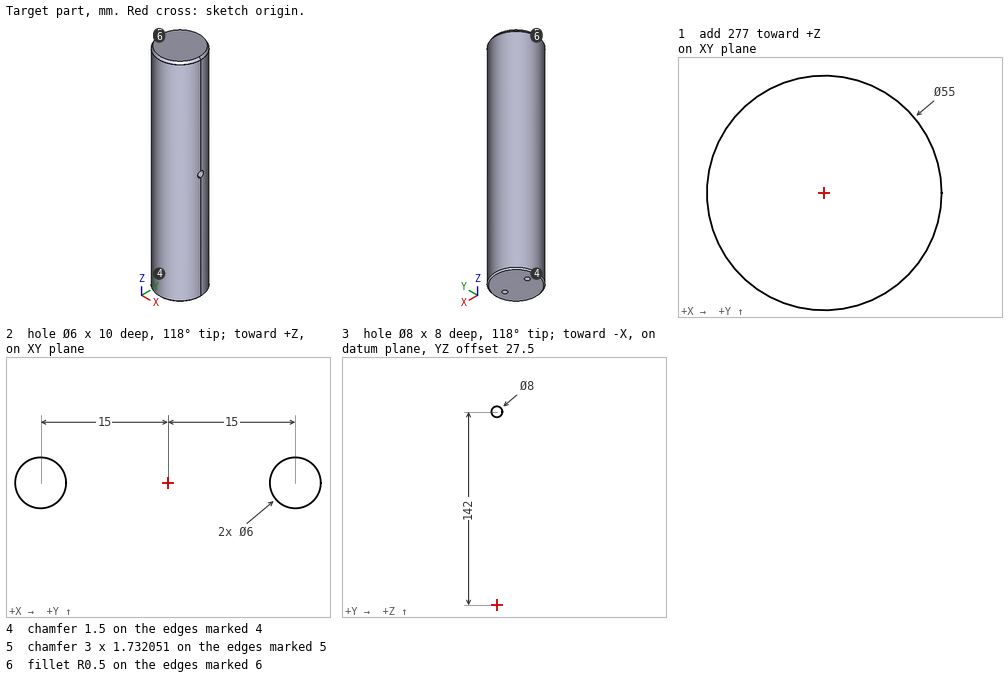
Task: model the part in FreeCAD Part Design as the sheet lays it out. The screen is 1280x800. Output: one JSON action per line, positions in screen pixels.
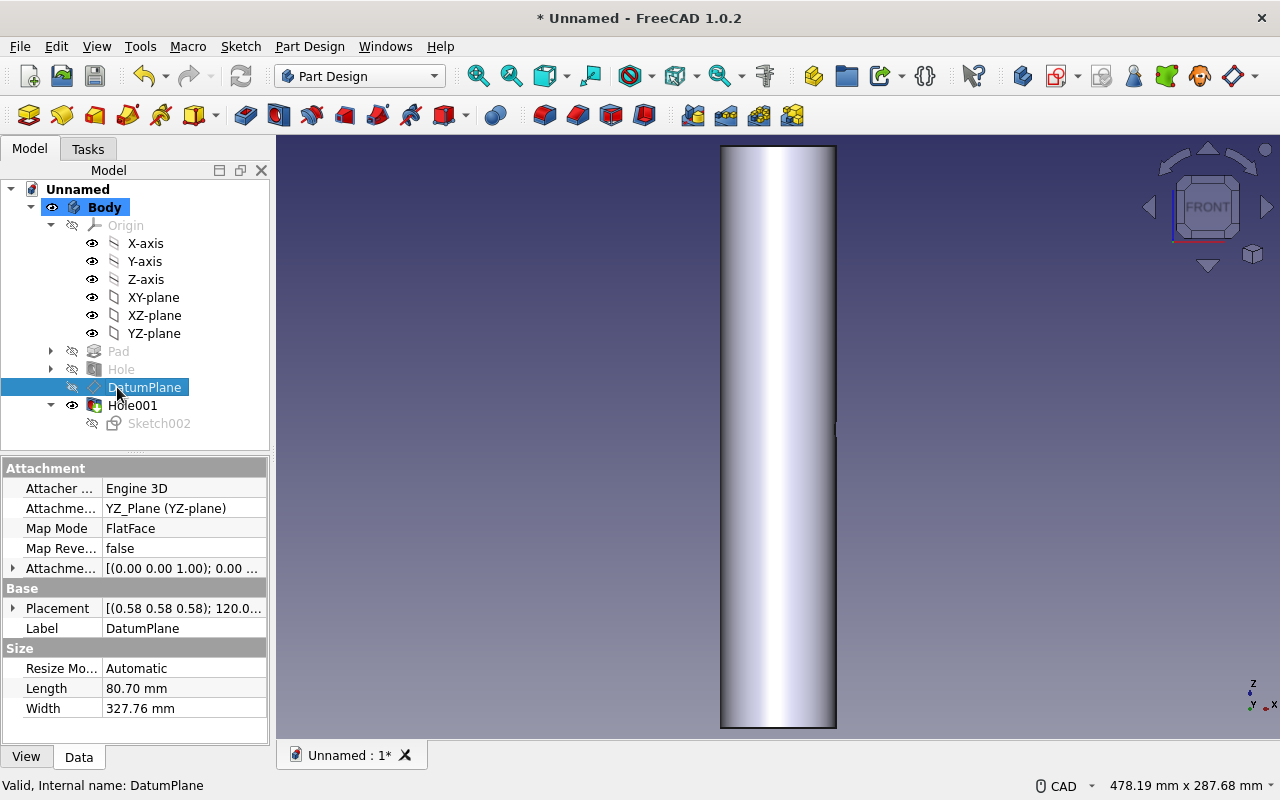
{"action": "key", "text": "3"}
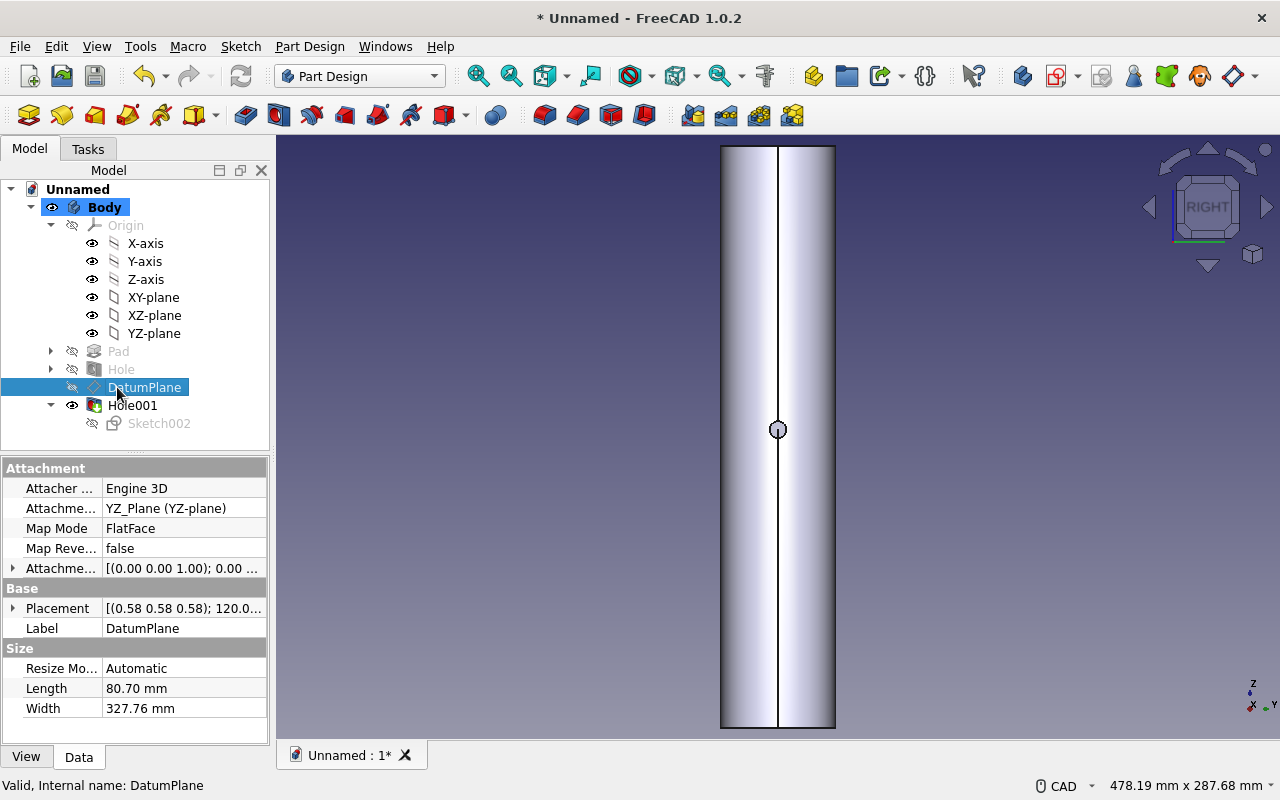
{"action": "key", "text": "5"}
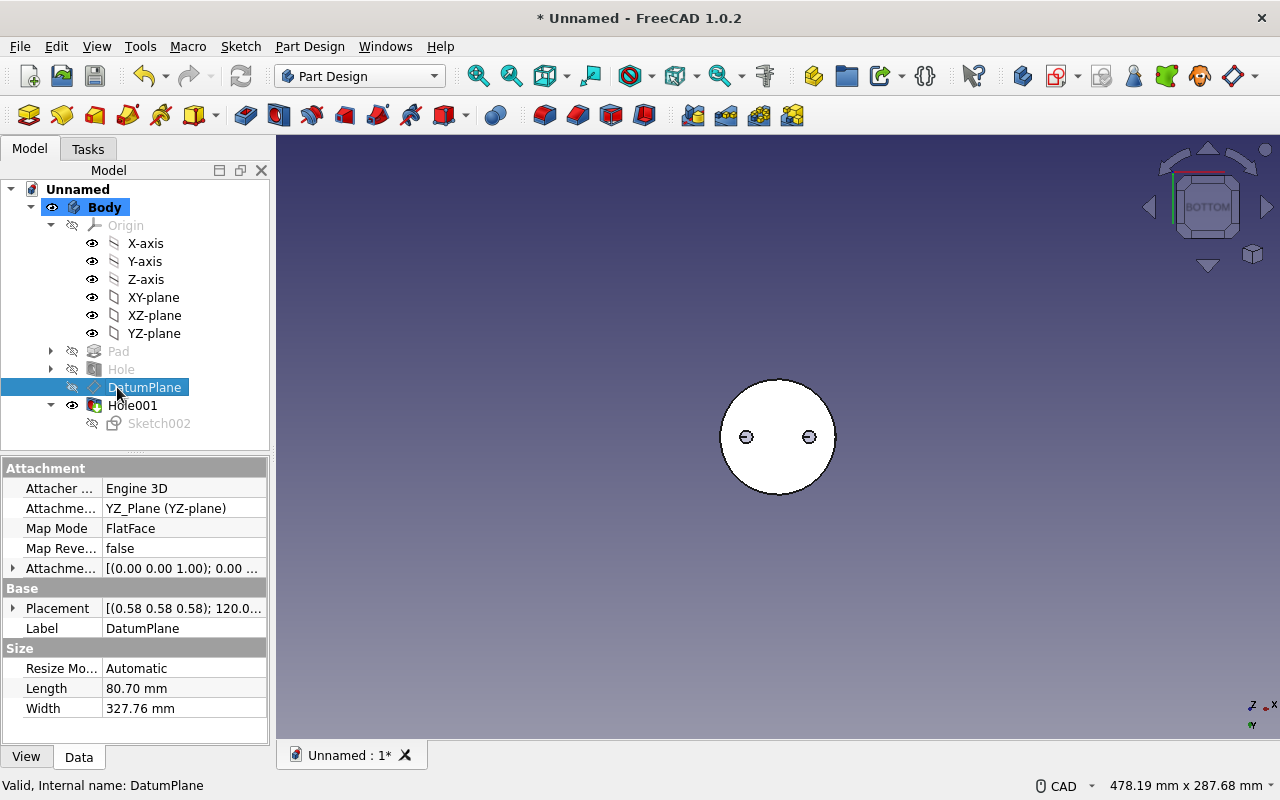
{"action": "left_click", "coordinate": [479, 76]}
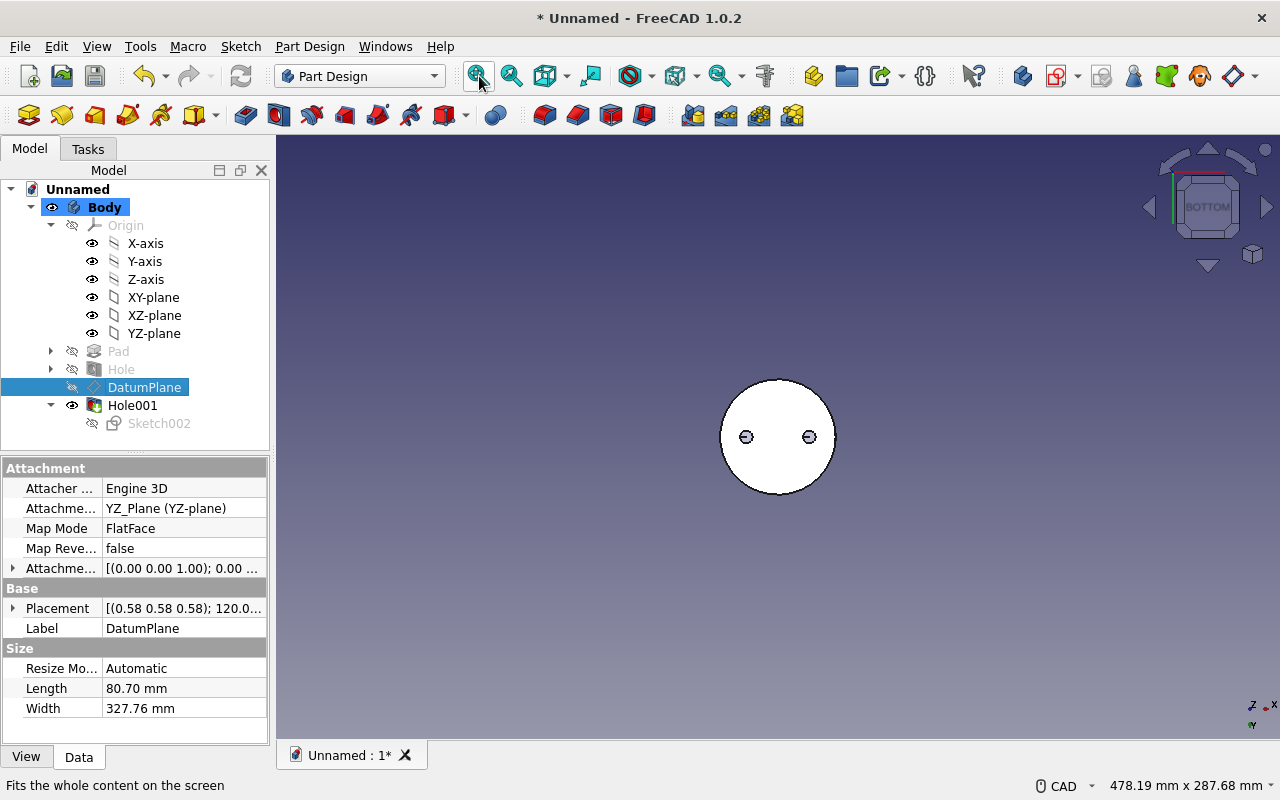
{"action": "left_click", "coordinate": [731, 470]}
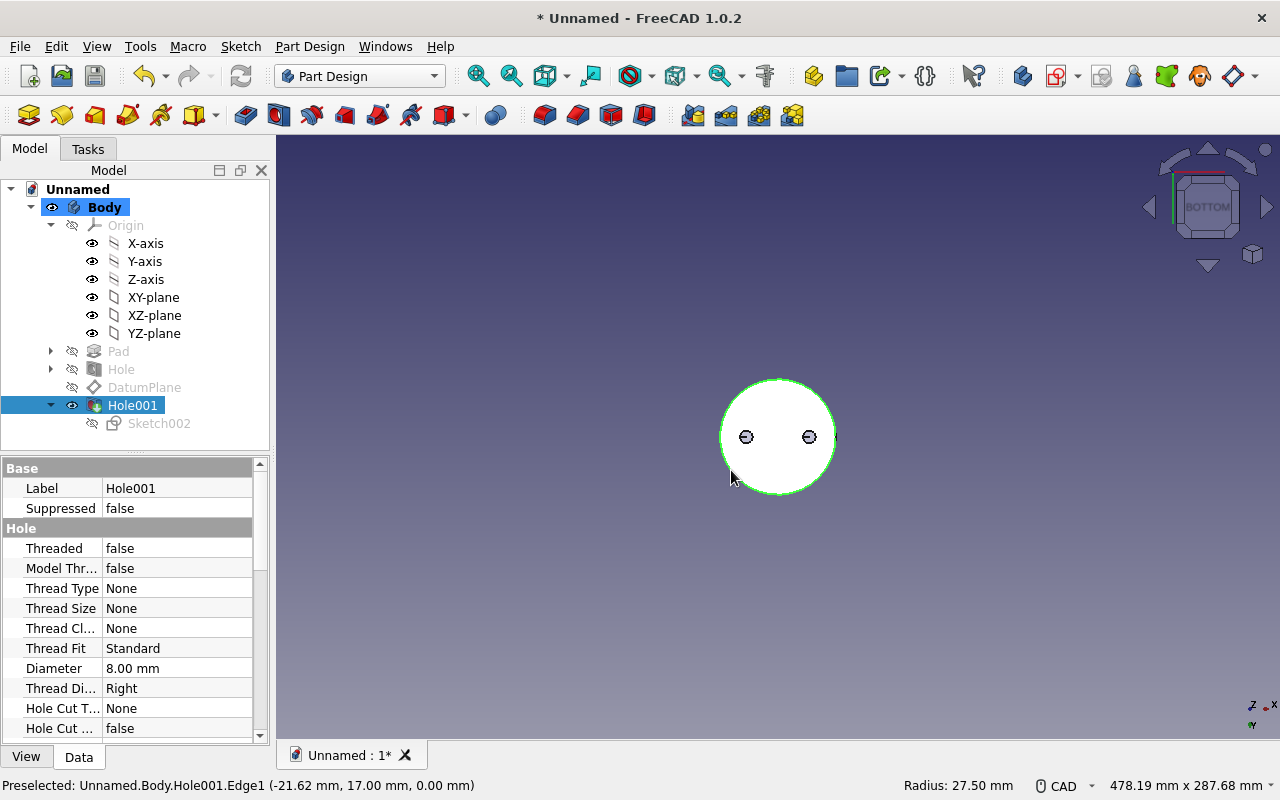
{"action": "left_click", "coordinate": [578, 116]}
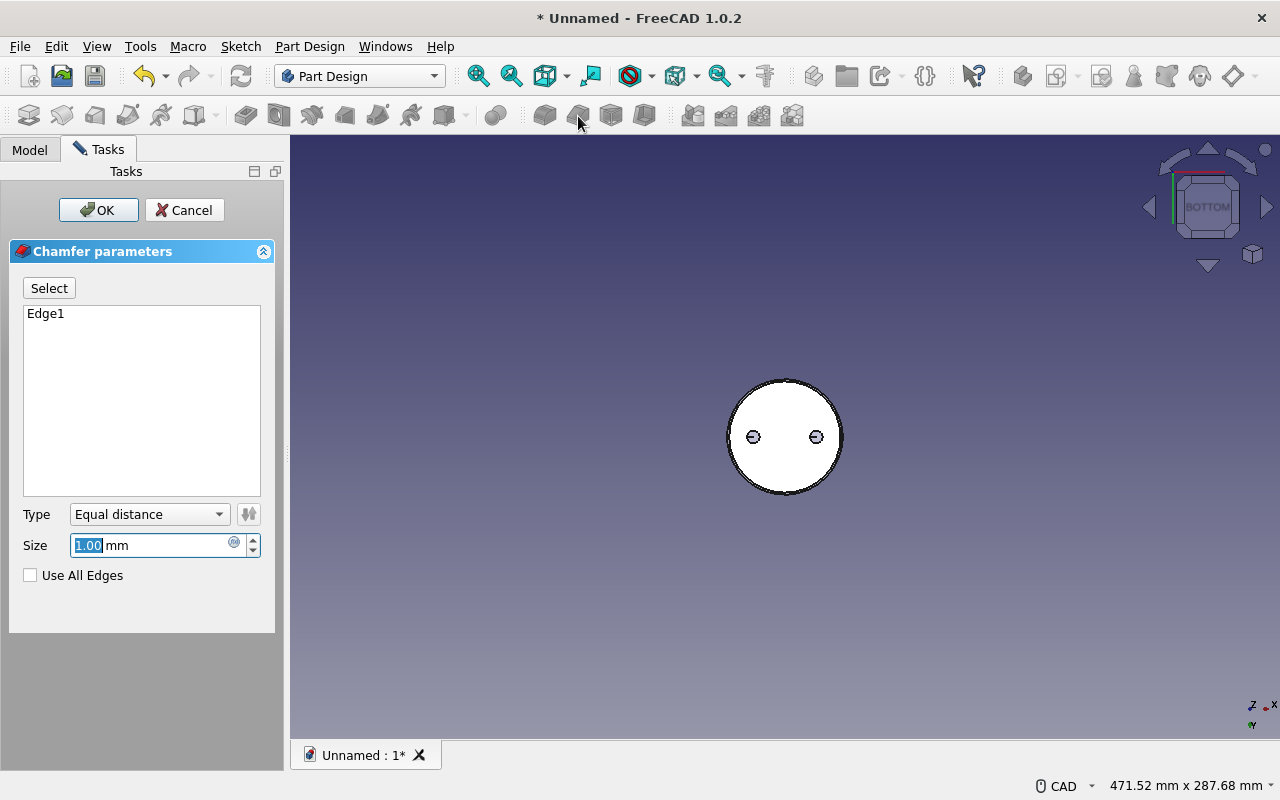
{"action": "type", "text": "1.5"}
{"action": "key", "text": "Tab"}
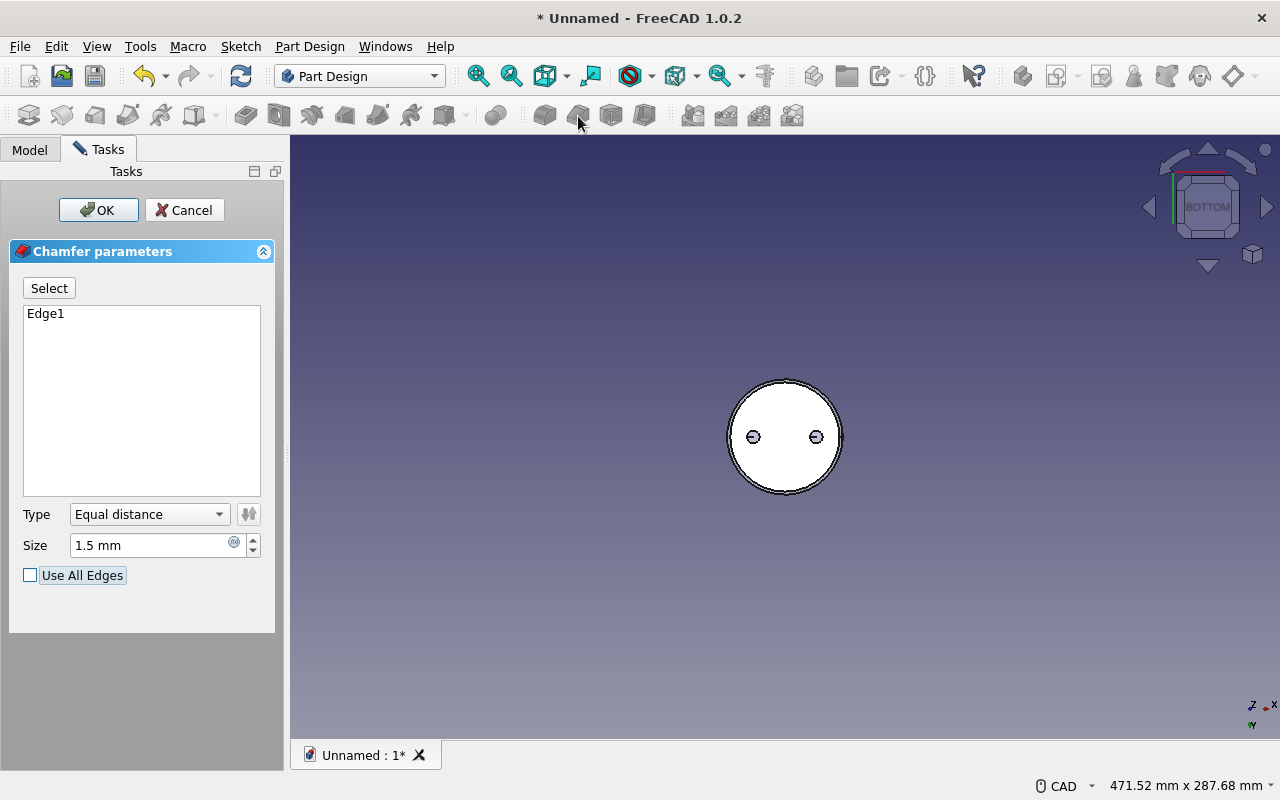
{"action": "left_click", "coordinate": [99, 210]}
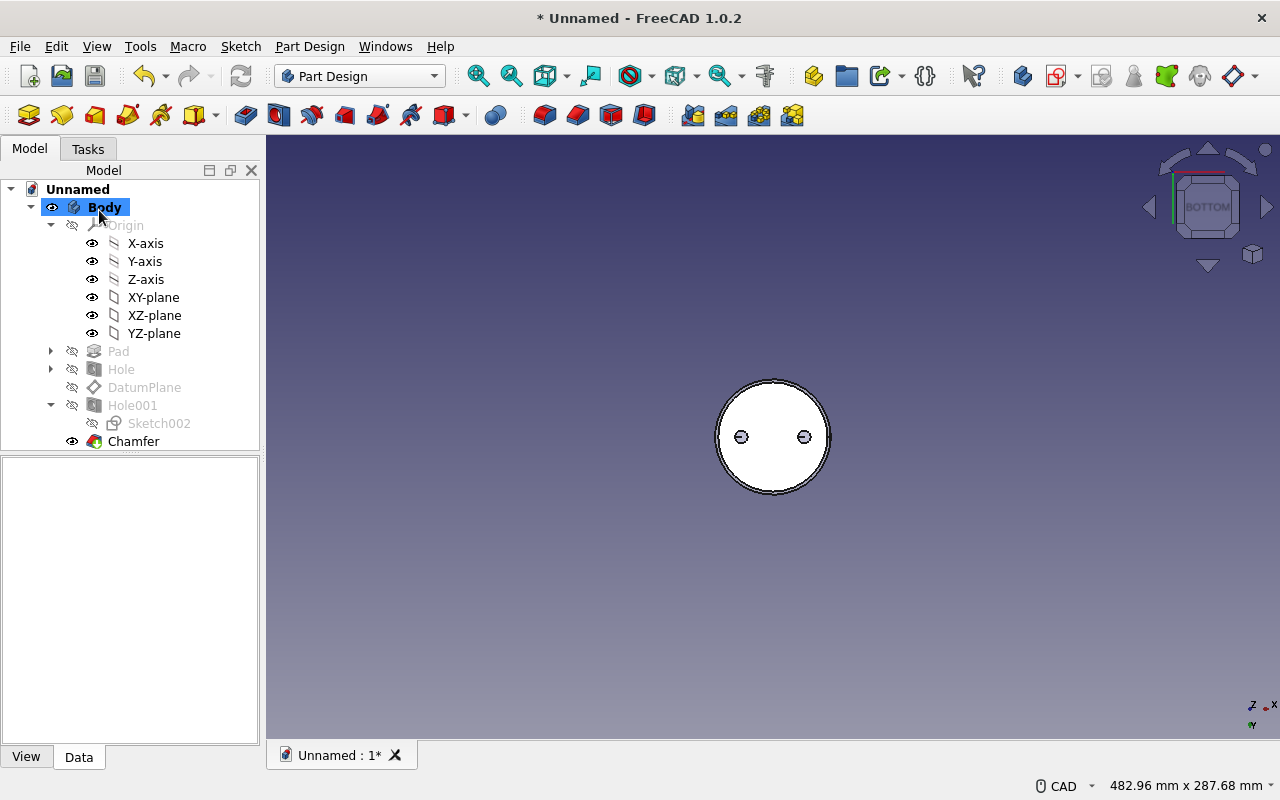
{"action": "key", "text": "v f"}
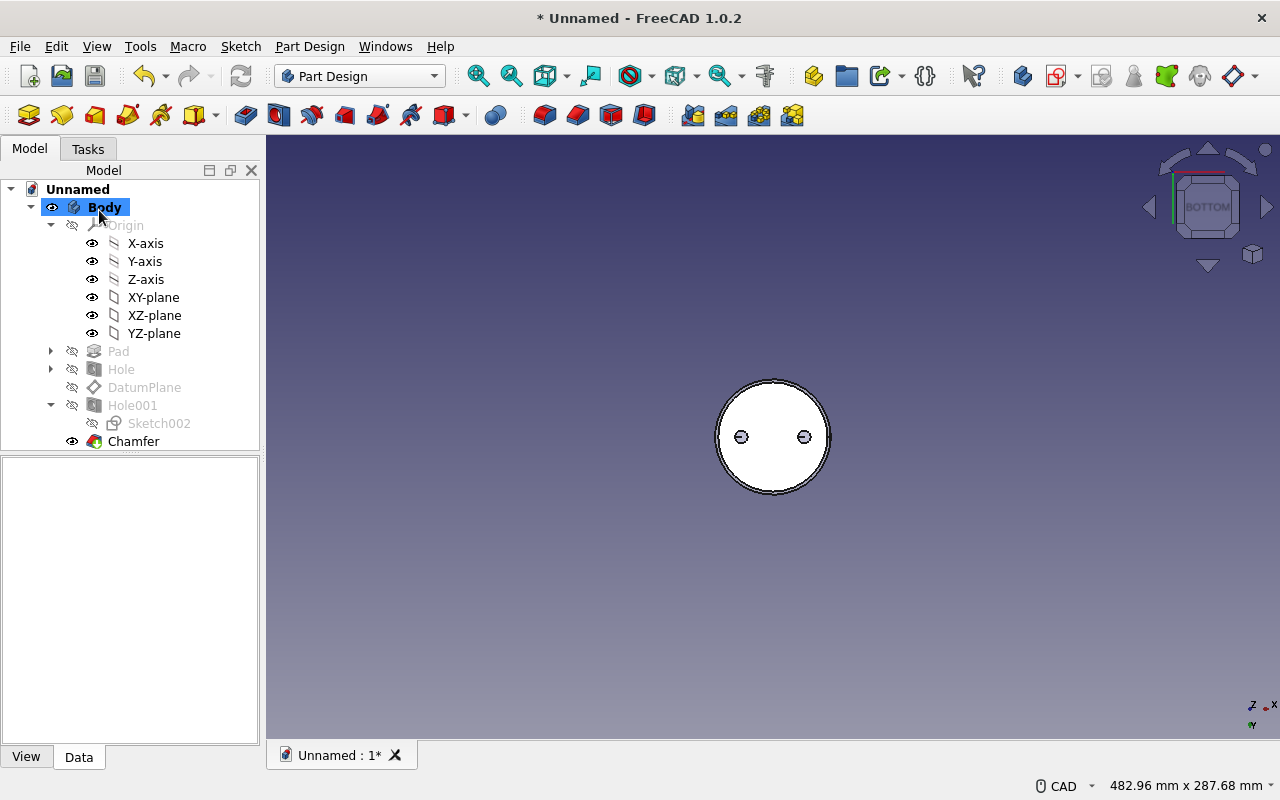
{"action": "key", "text": "0"}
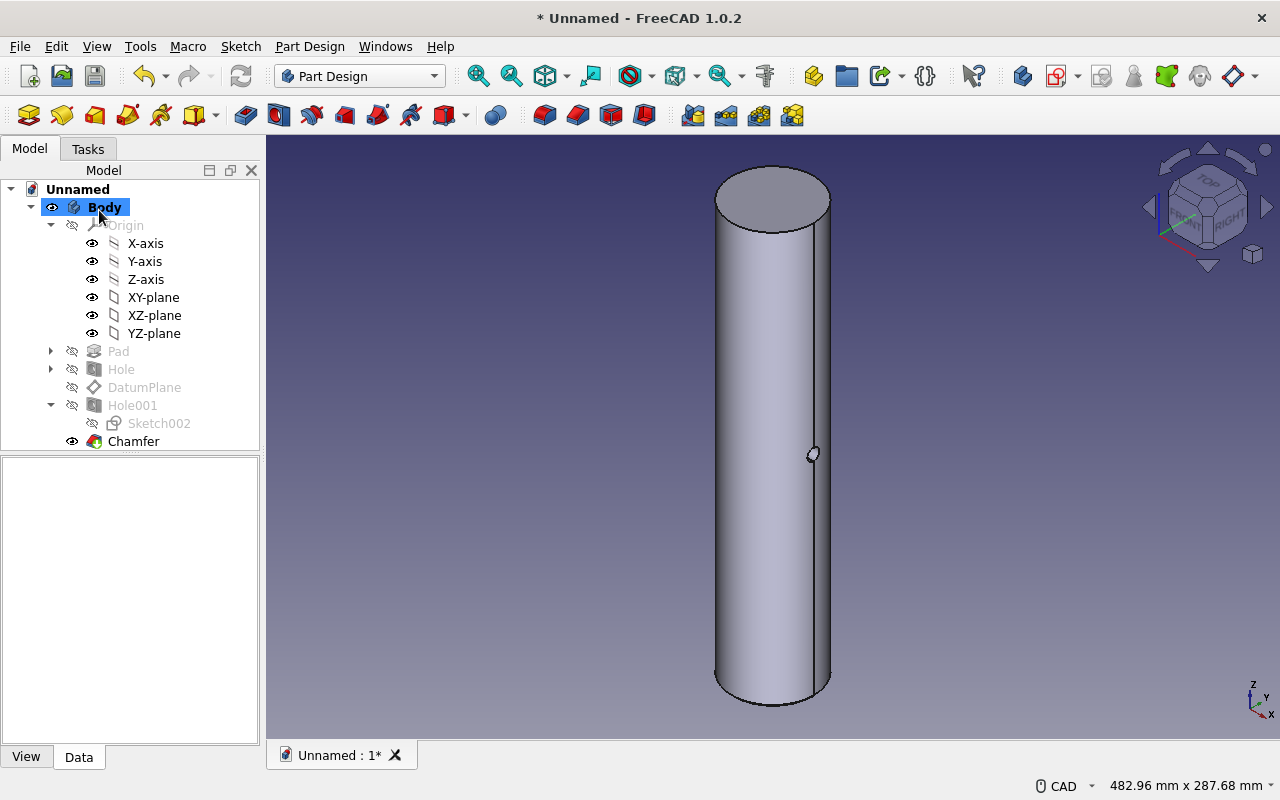
{"action": "left_click", "coordinate": [716, 193]}